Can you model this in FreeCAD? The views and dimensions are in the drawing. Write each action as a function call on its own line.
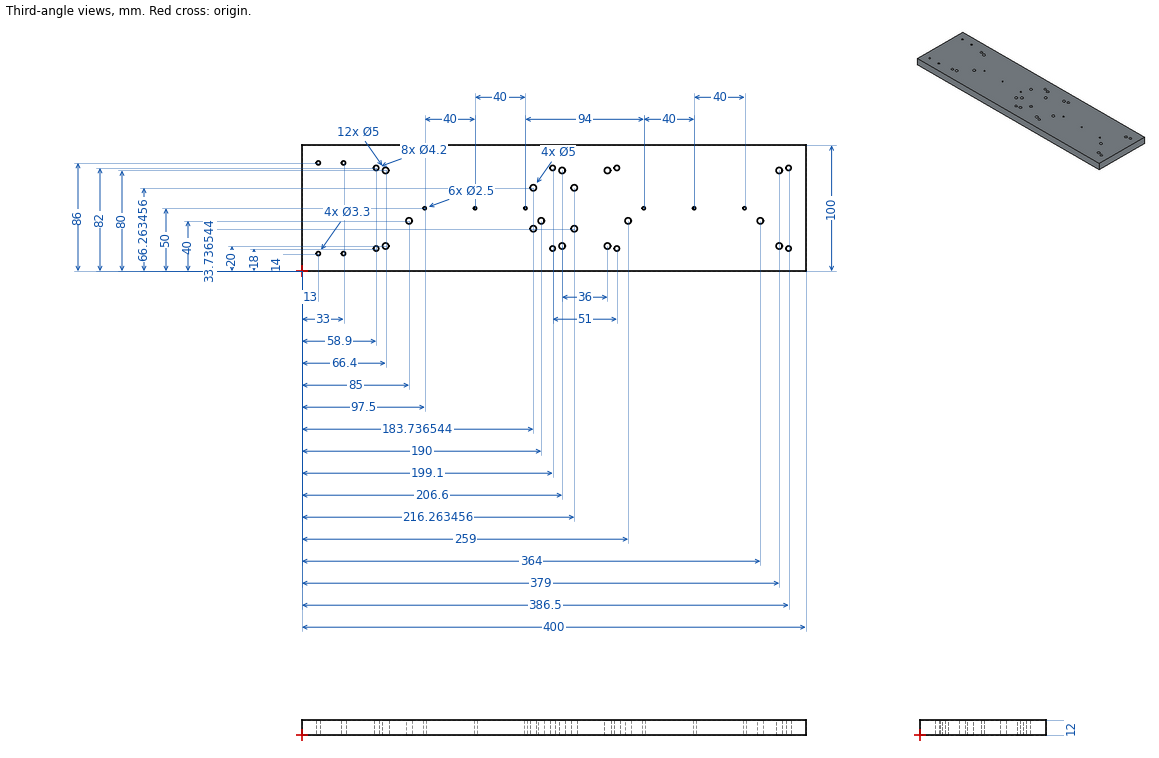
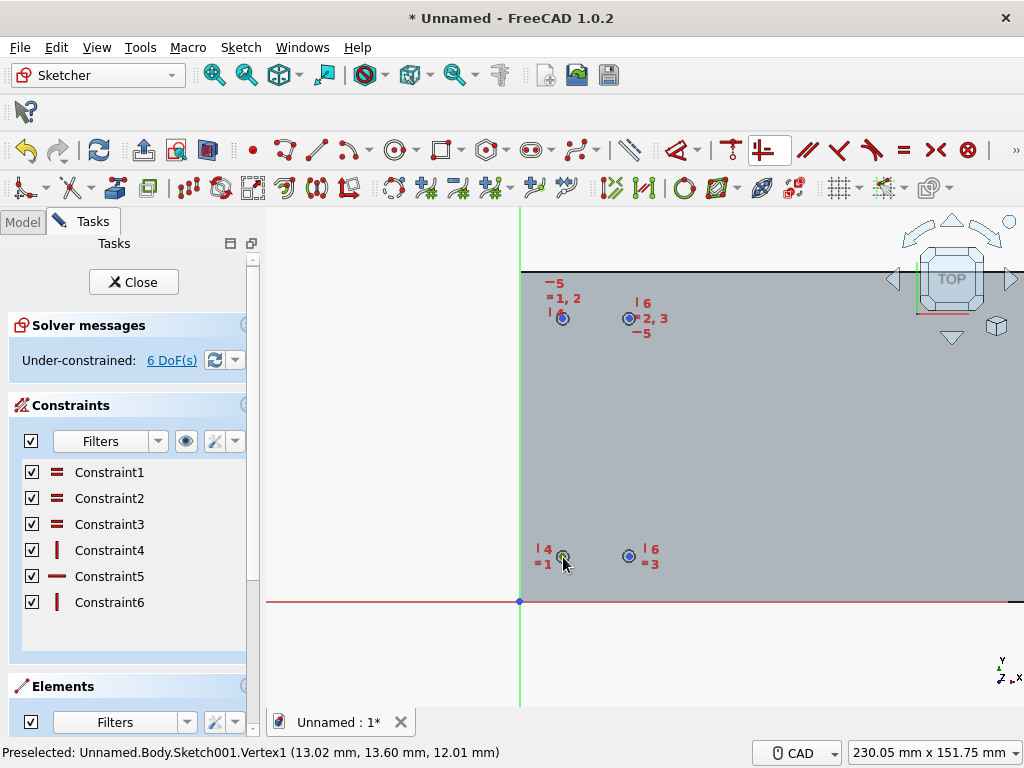
click(629, 556)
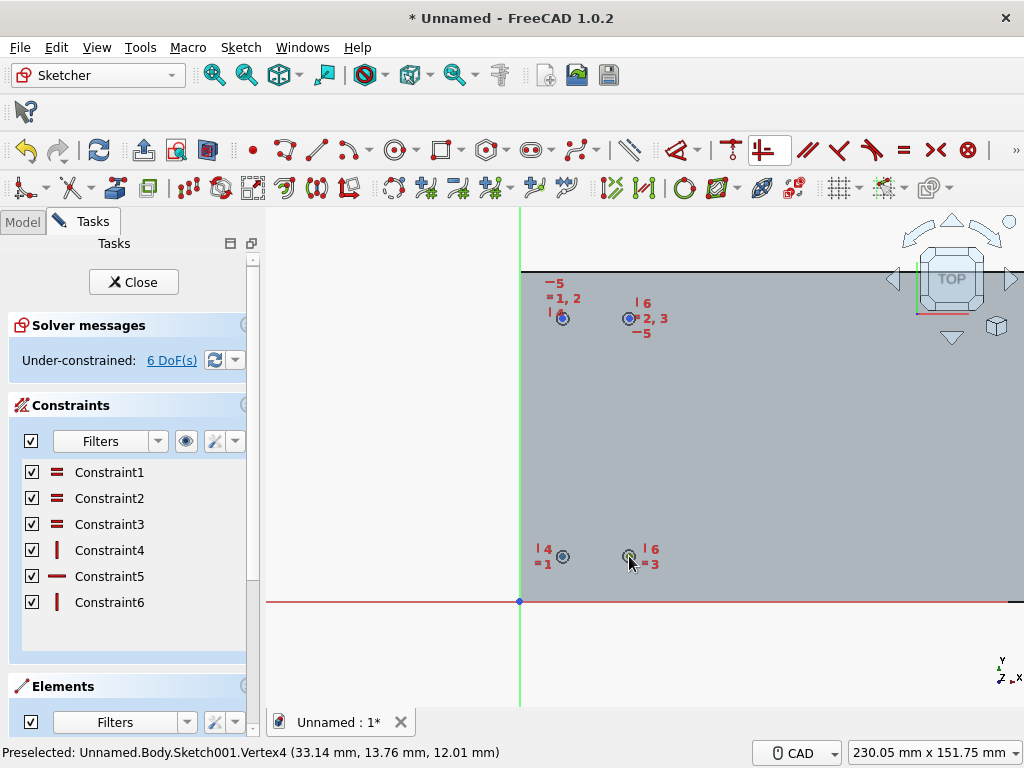
click(786, 150)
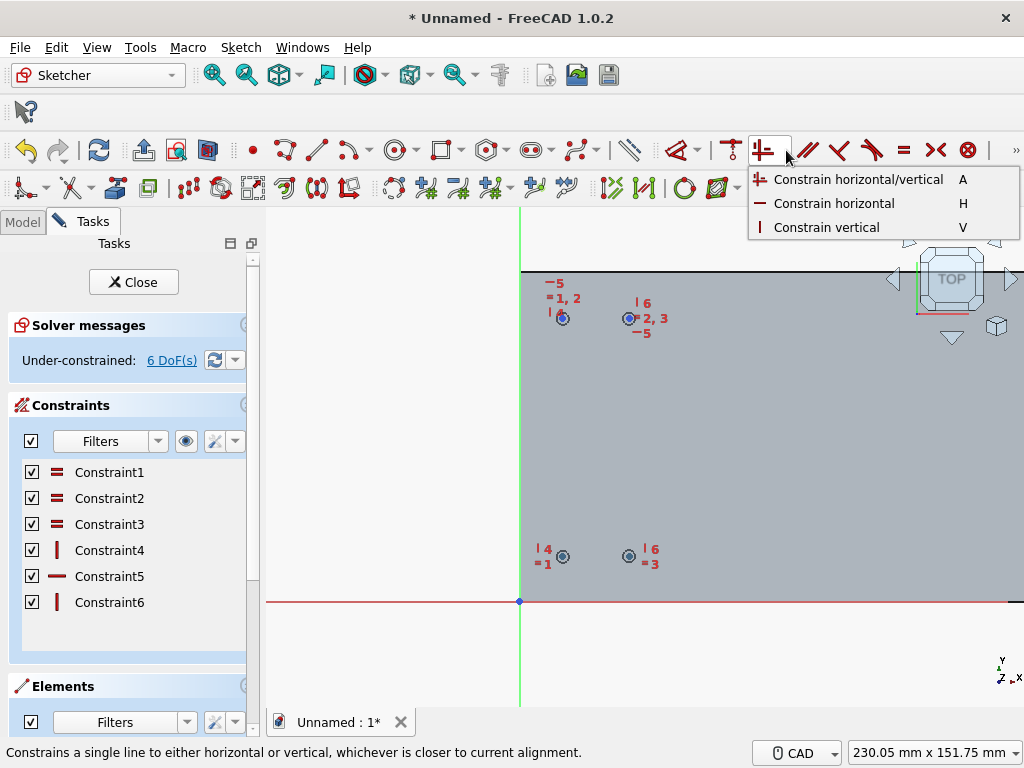
click(884, 203)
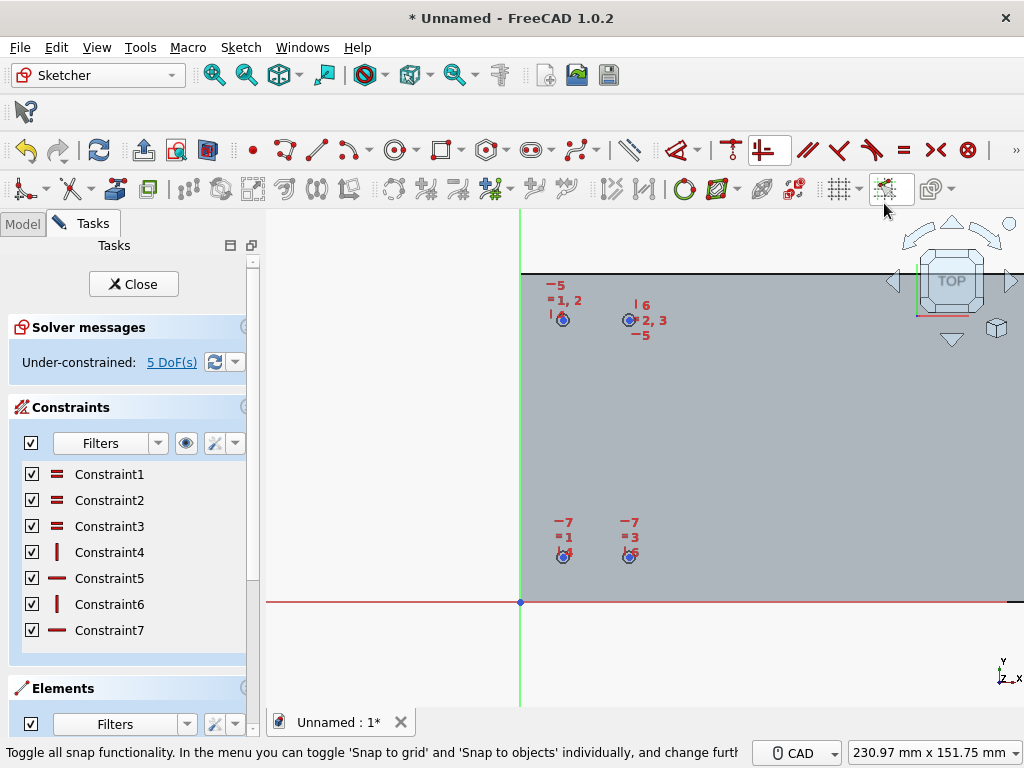
click(676, 150)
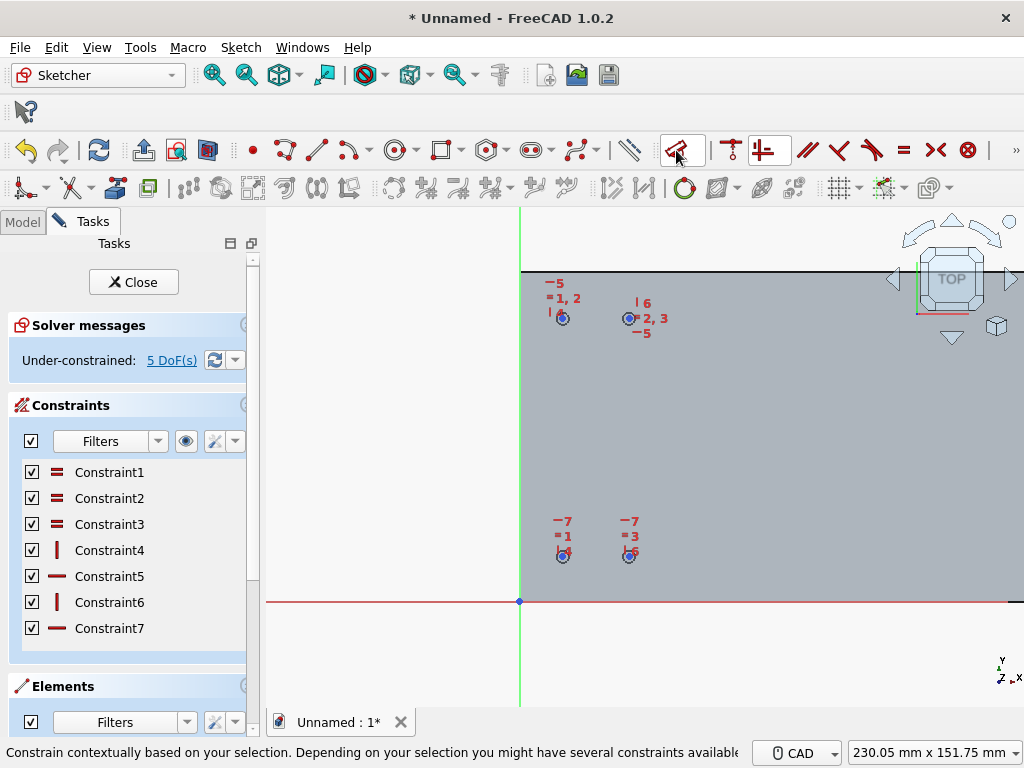
scroll(558, 553, up, 7)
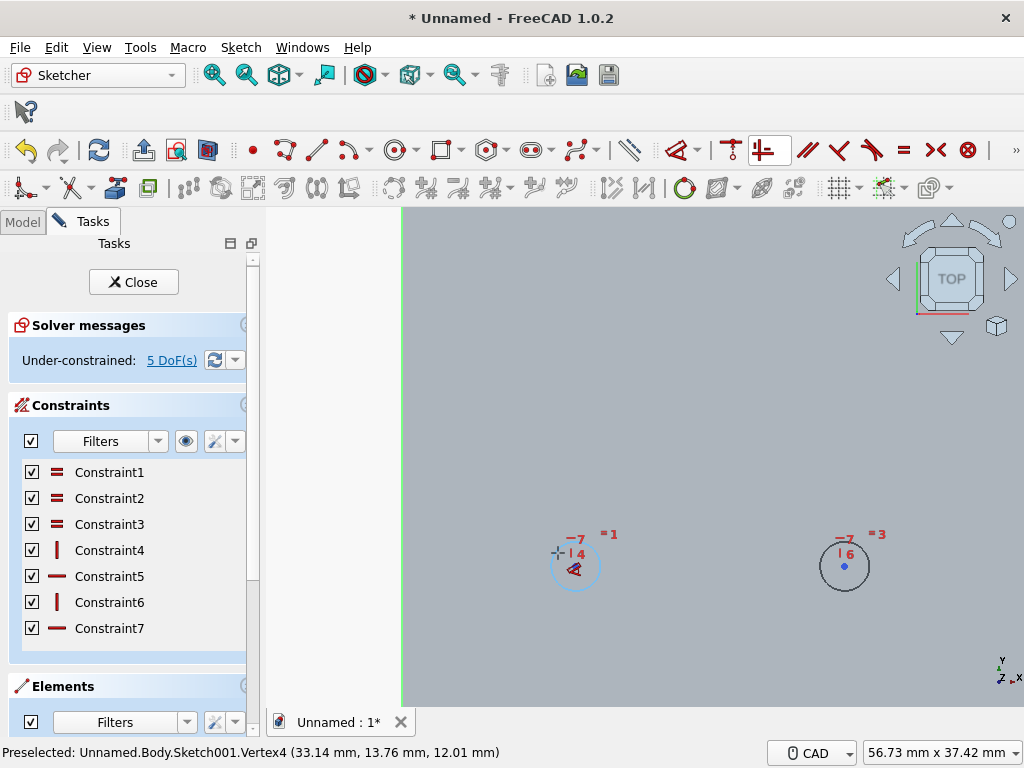
click(558, 549)
click(535, 527)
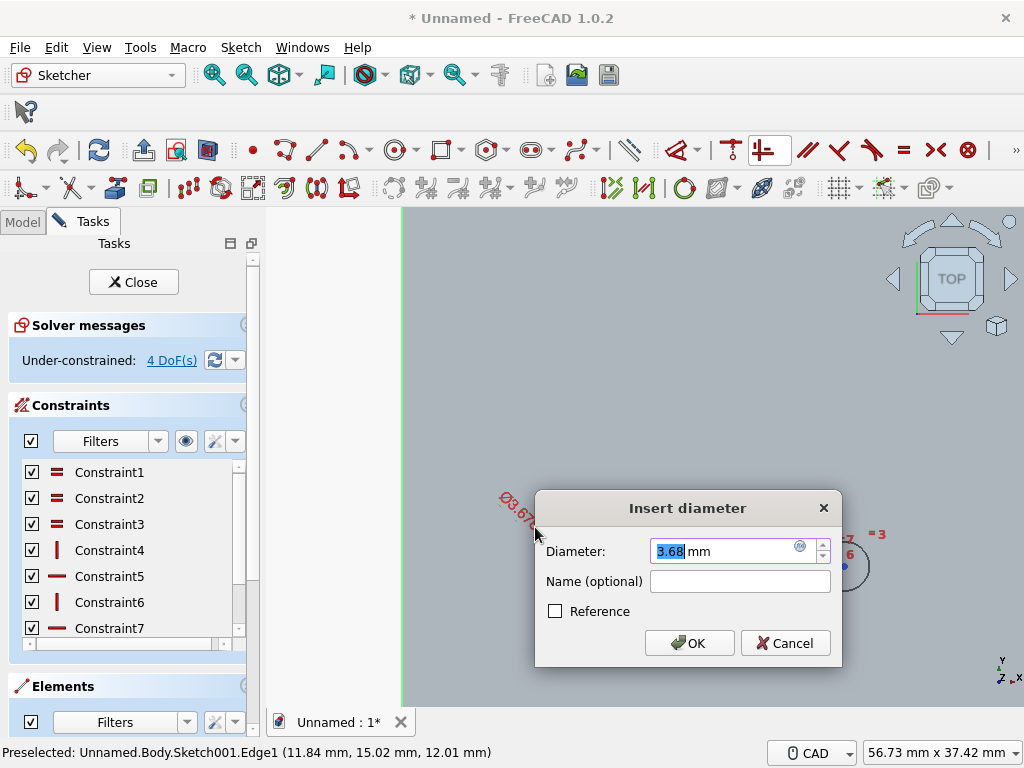
text(3.3)
key(Return)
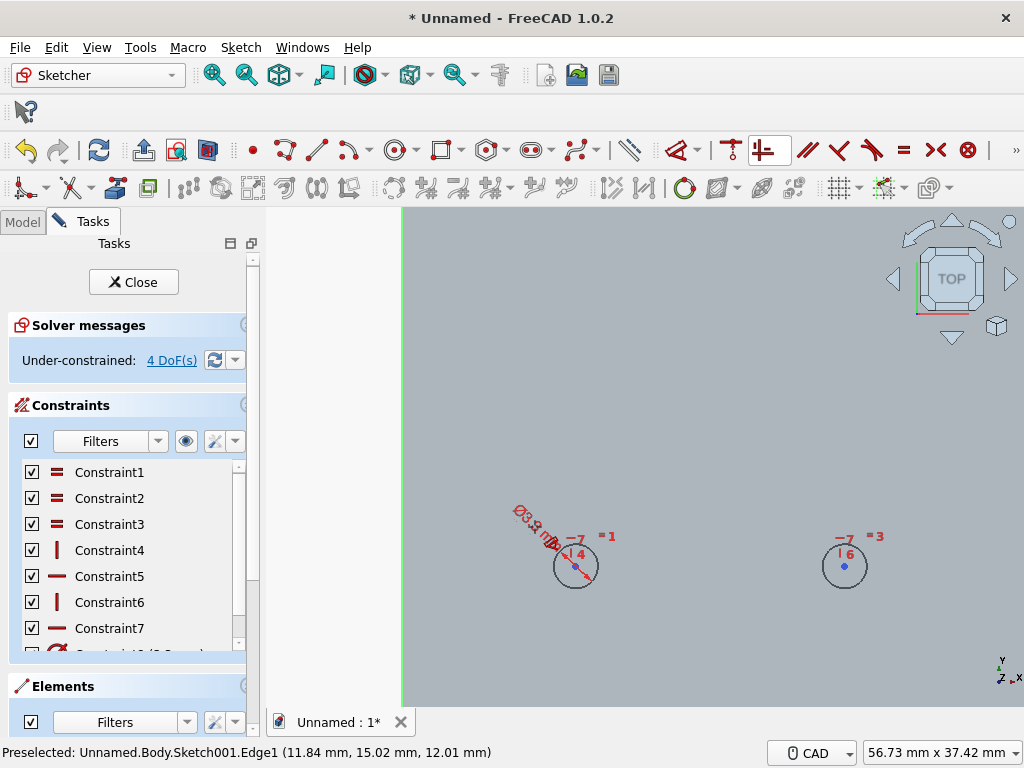
scroll(558, 553, down, 7)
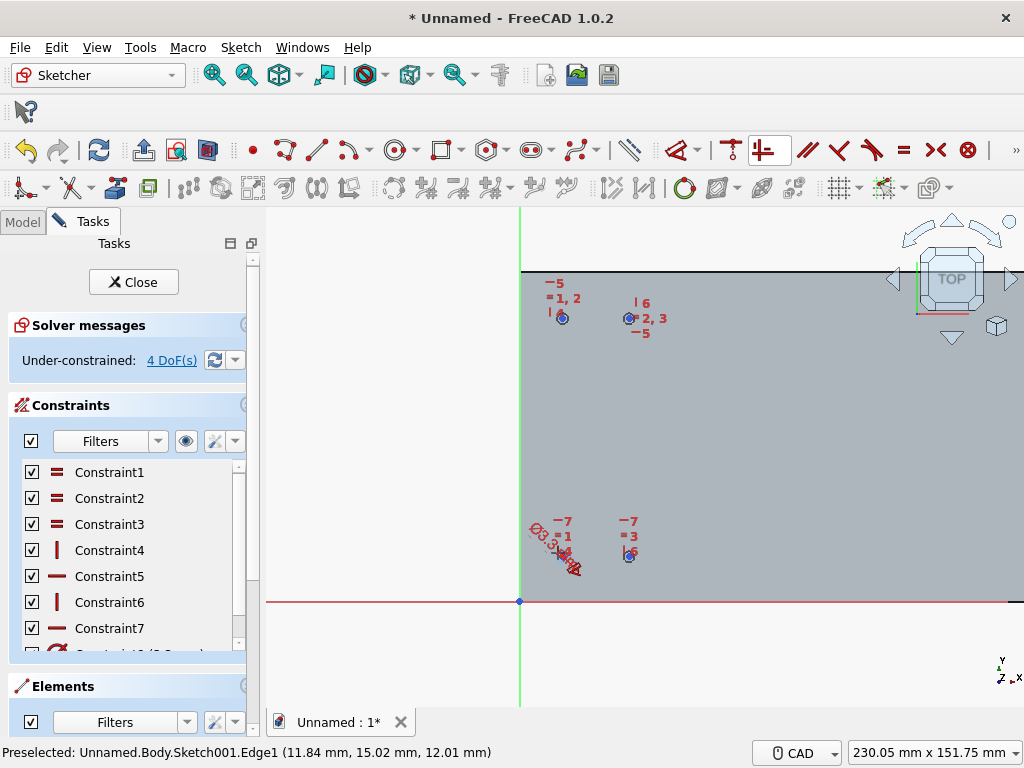
click(563, 557)
click(541, 636)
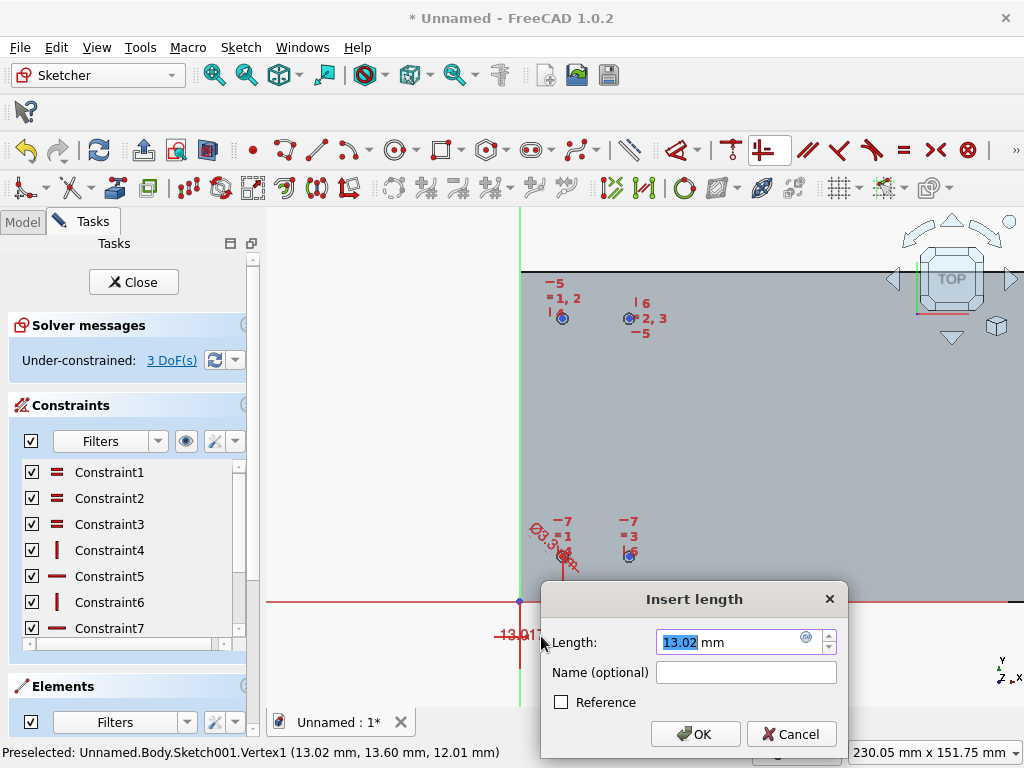
text(13)
key(Return)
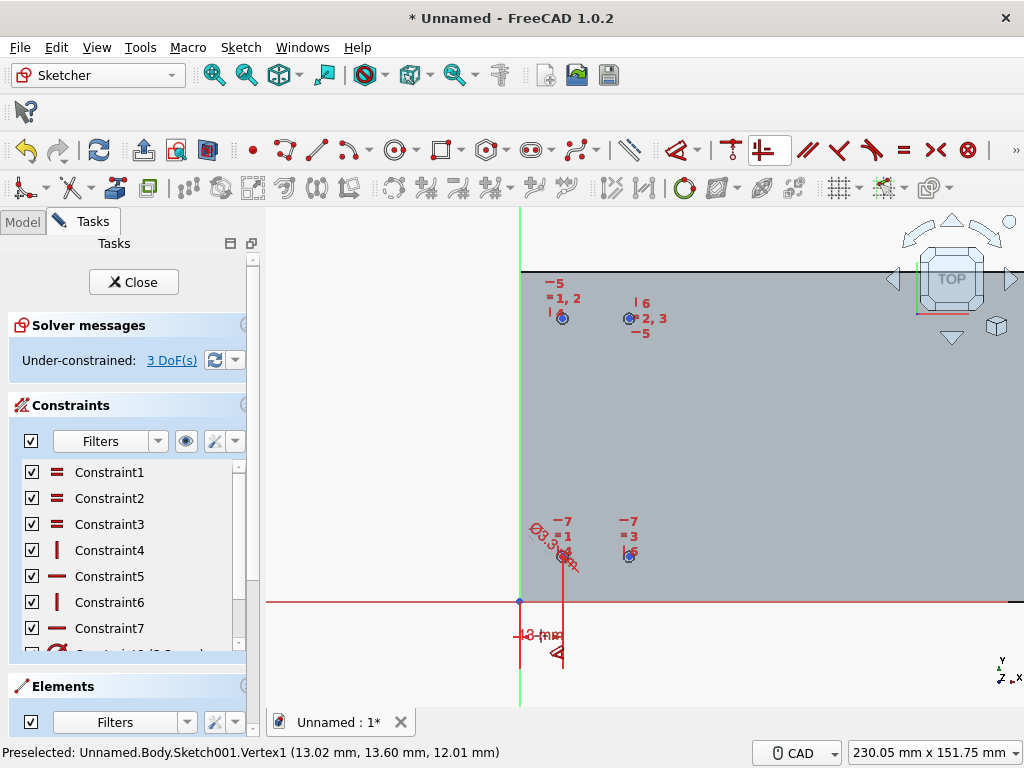
click(563, 557)
click(486, 579)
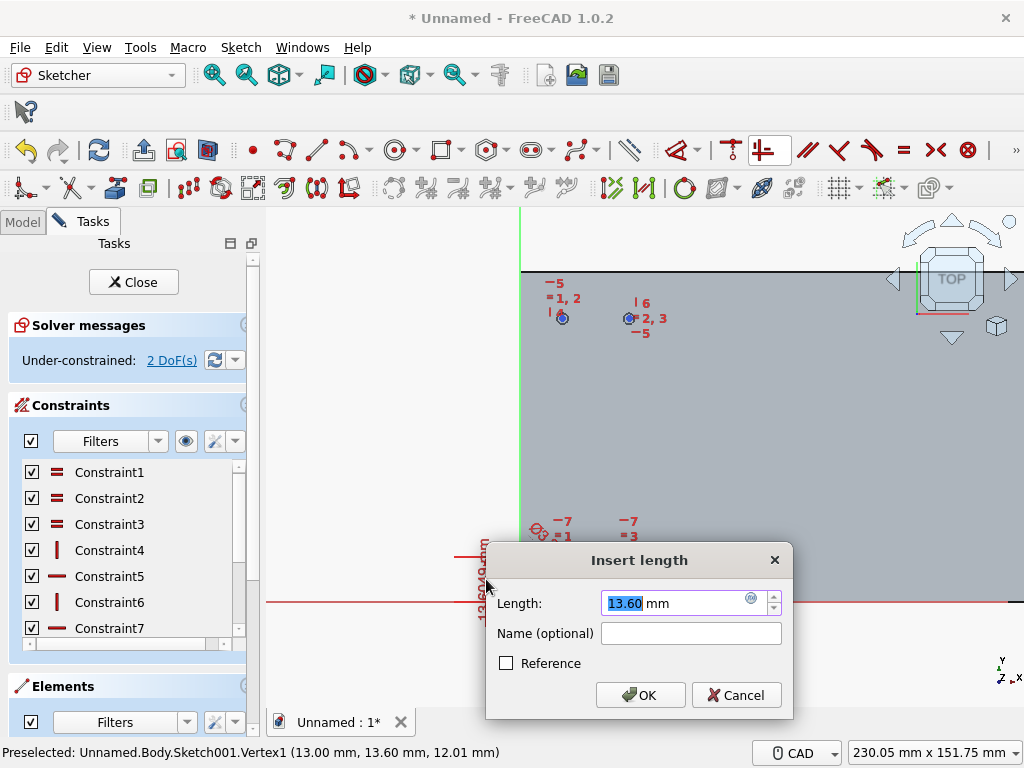
text(14)
key(Return)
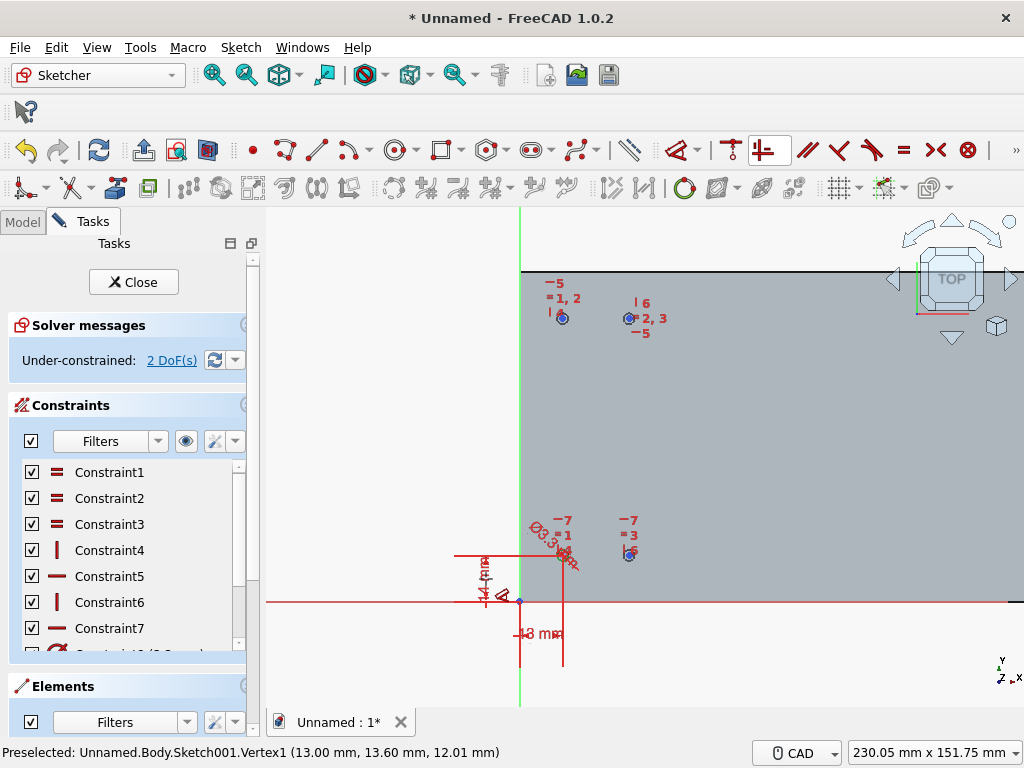
click(563, 319)
click(486, 460)